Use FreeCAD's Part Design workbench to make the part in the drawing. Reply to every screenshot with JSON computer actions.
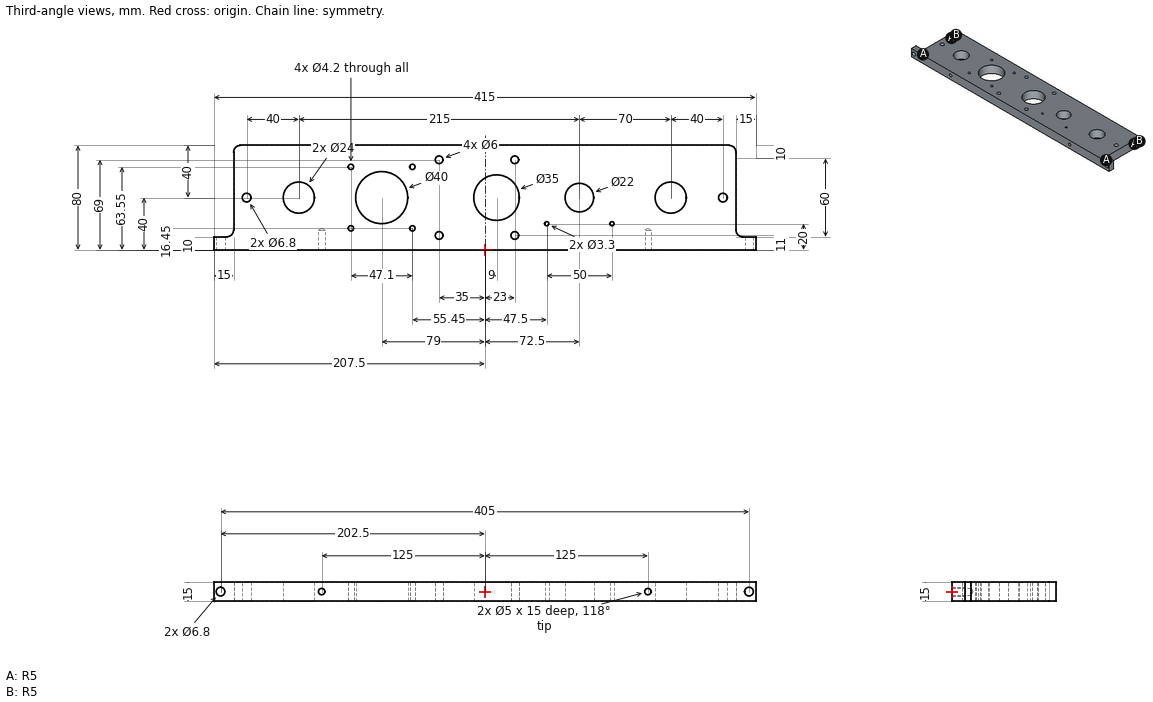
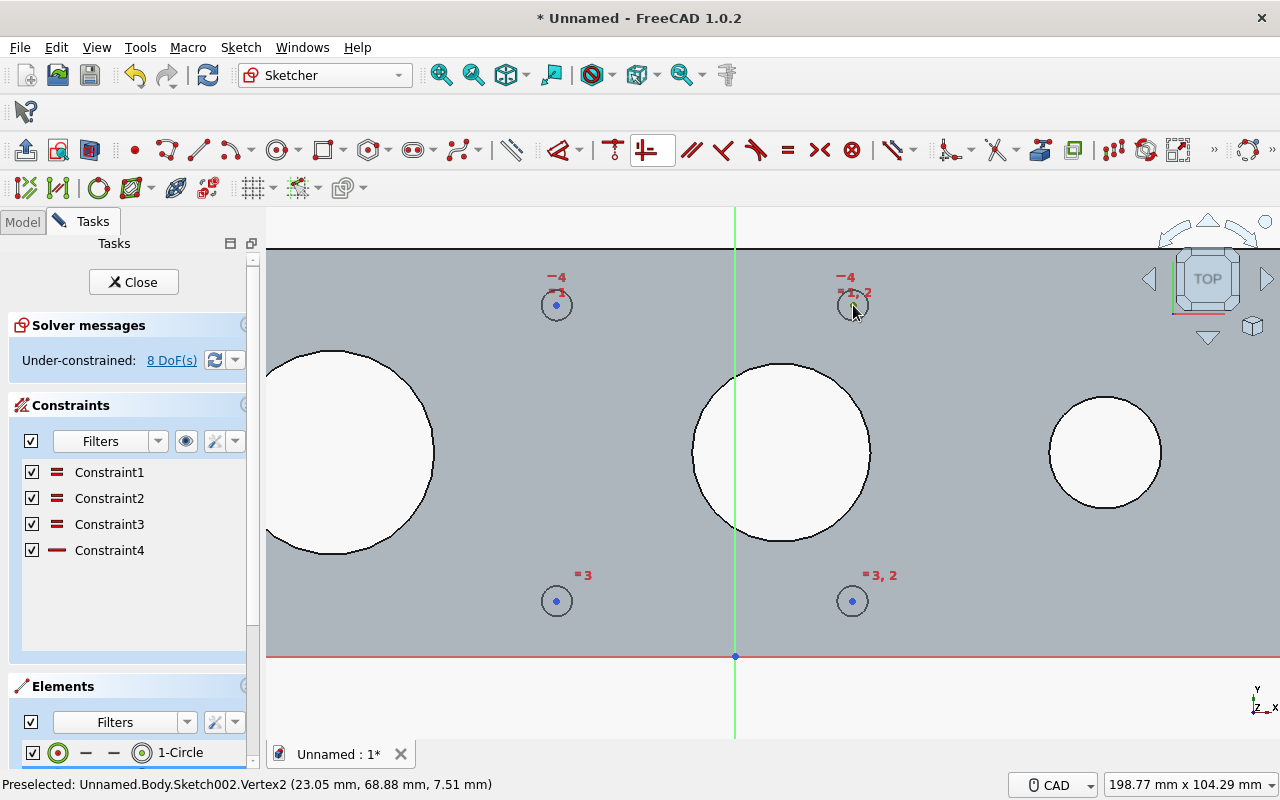
{"action": "left_click", "coordinate": [853, 601]}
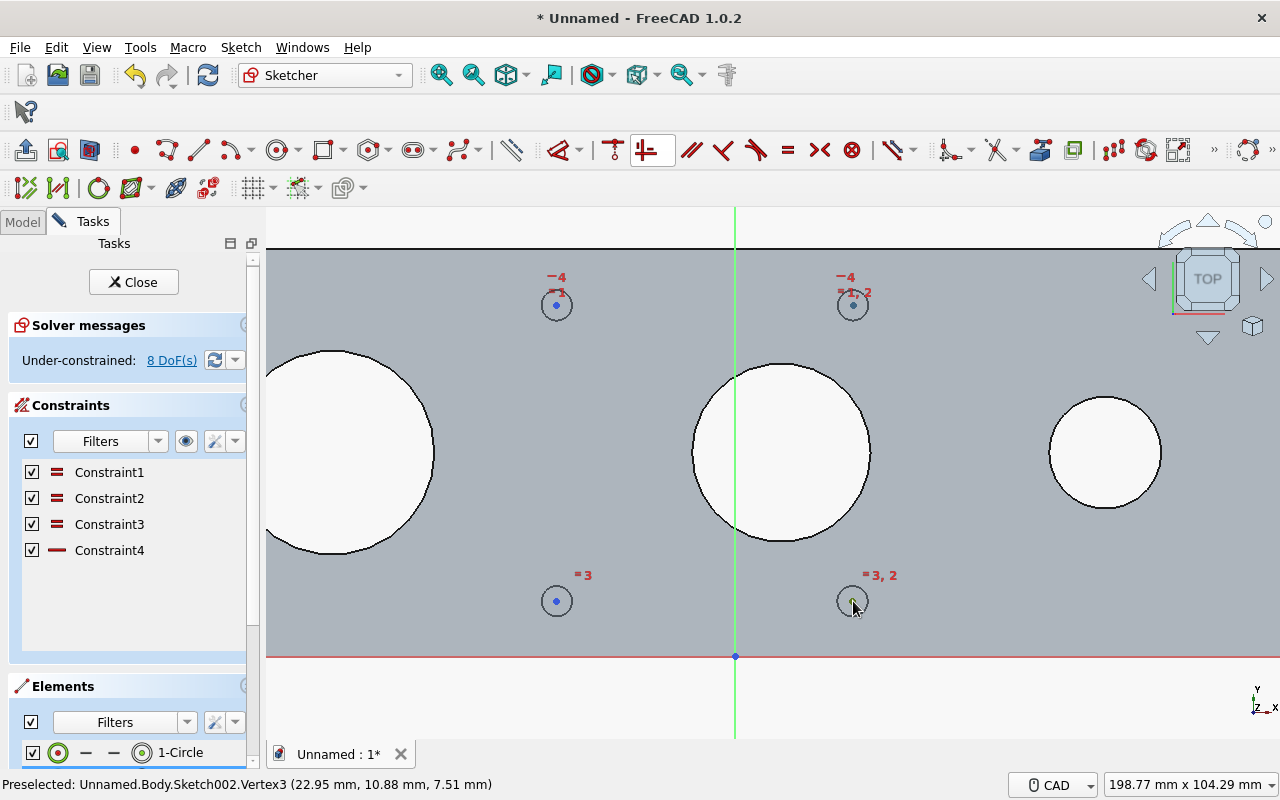
{"action": "left_click", "coordinate": [670, 150]}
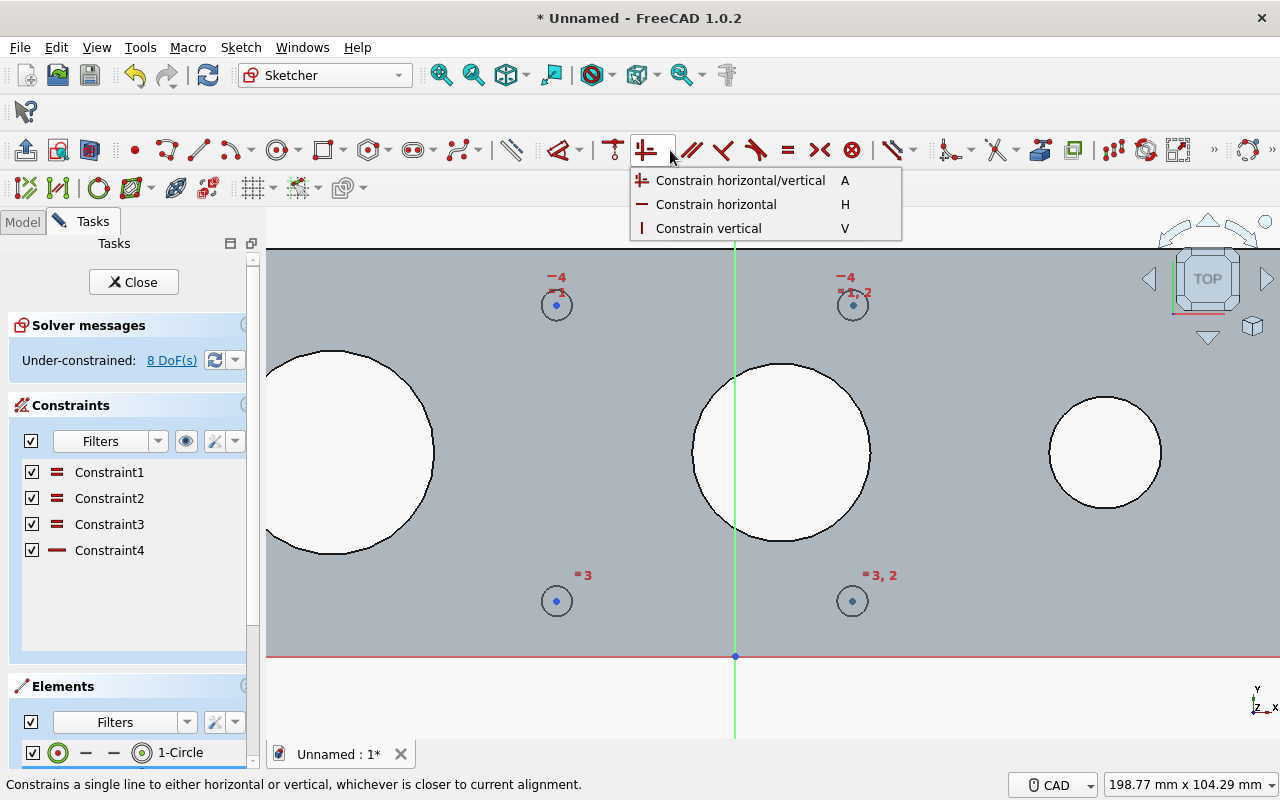
{"action": "left_click", "coordinate": [766, 228]}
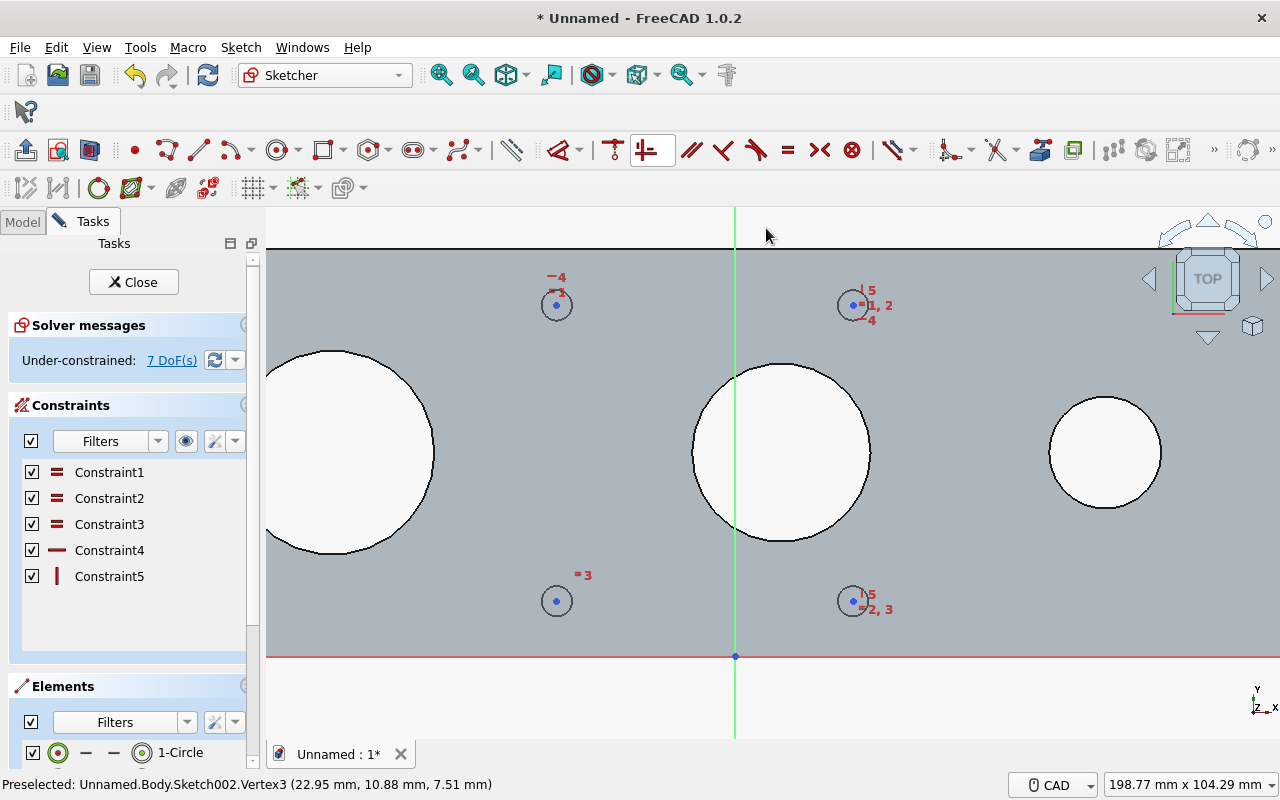
{"action": "left_click", "coordinate": [557, 305]}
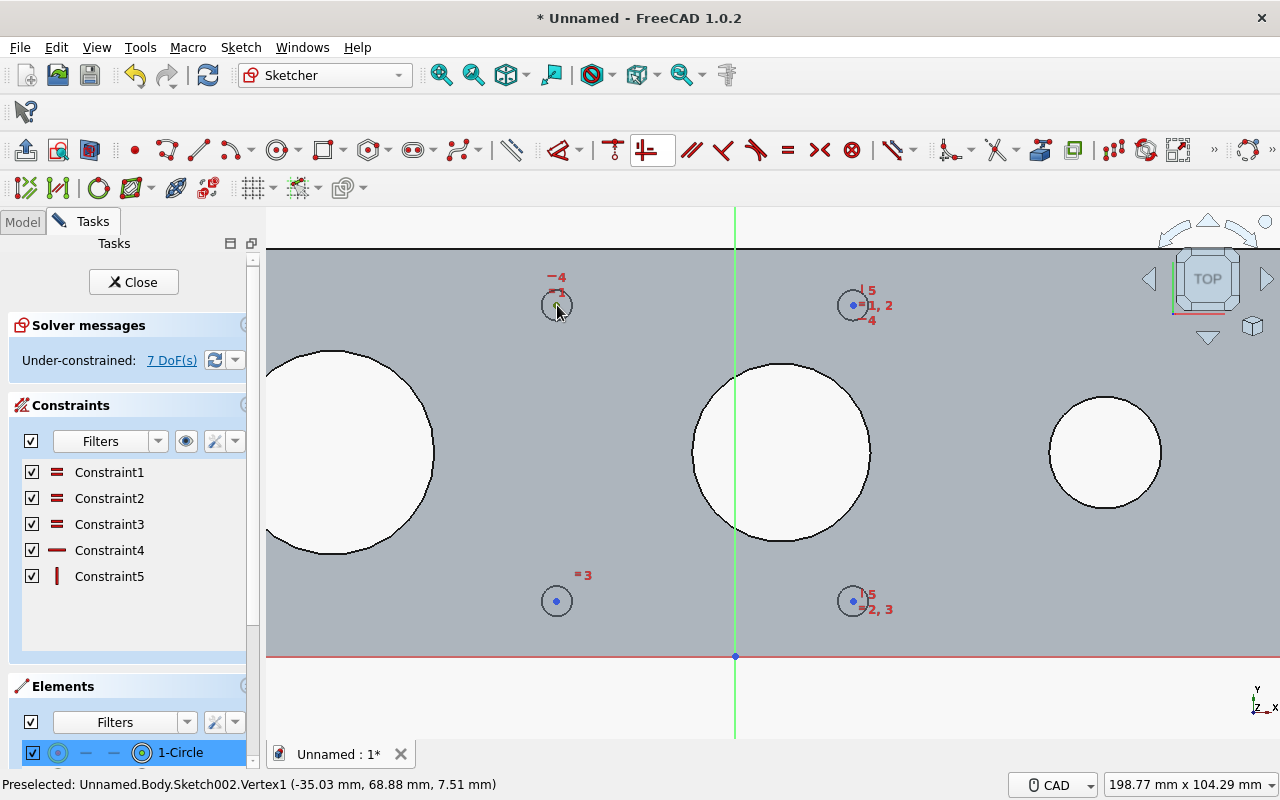
{"action": "left_click", "coordinate": [557, 601]}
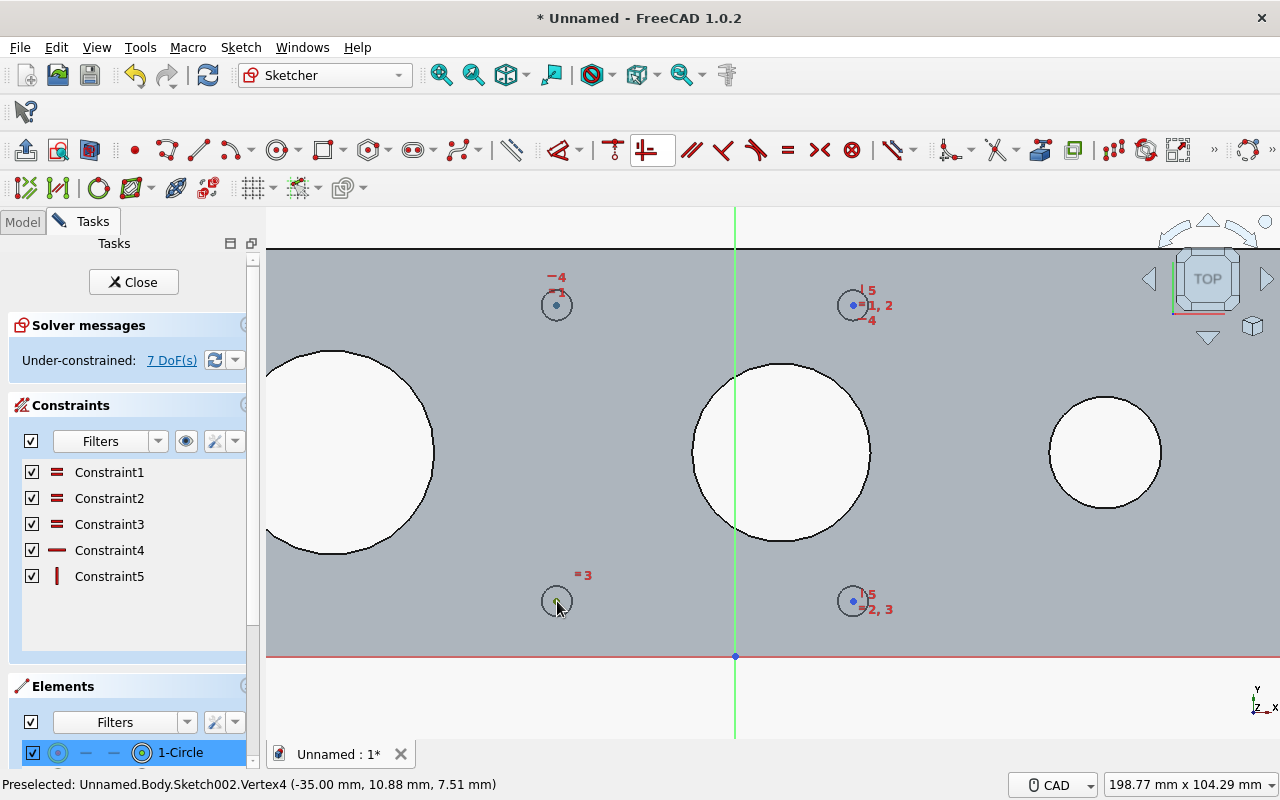
{"action": "key", "text": "v"}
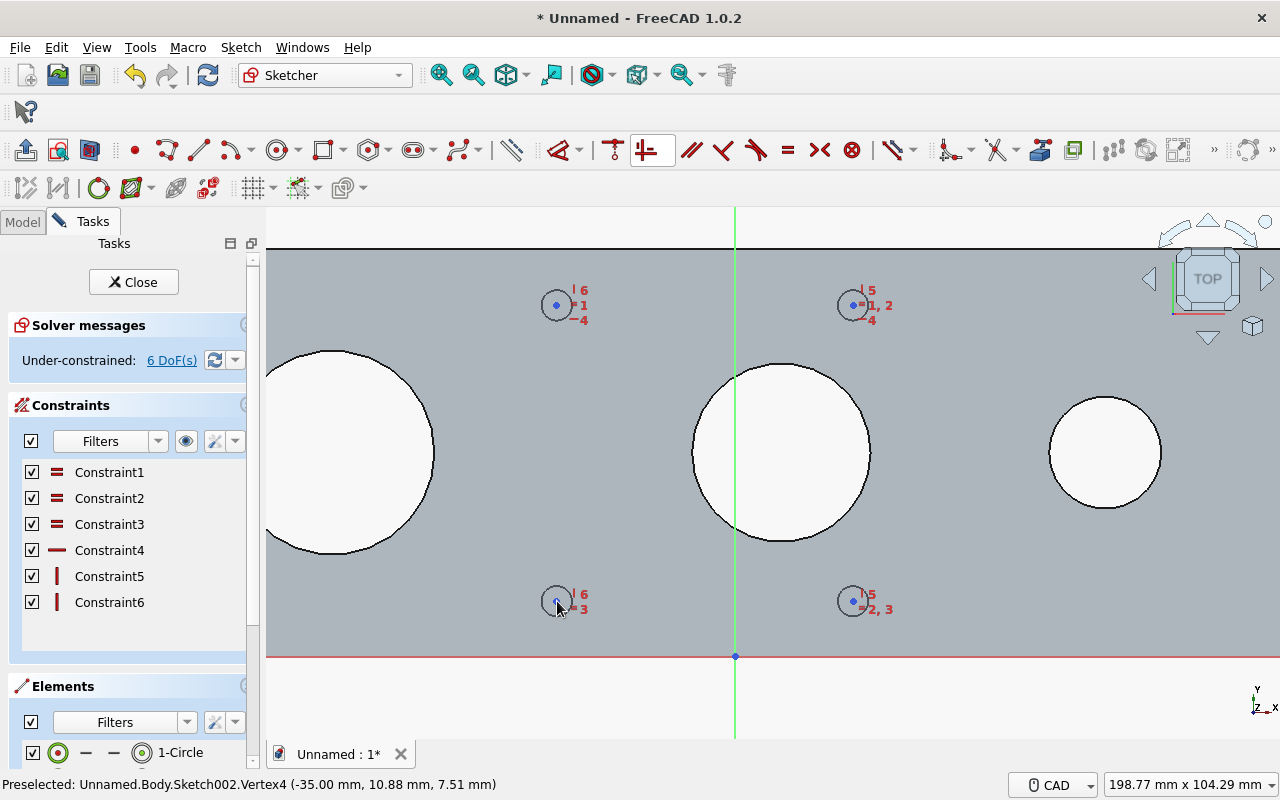
{"action": "left_click", "coordinate": [853, 601]}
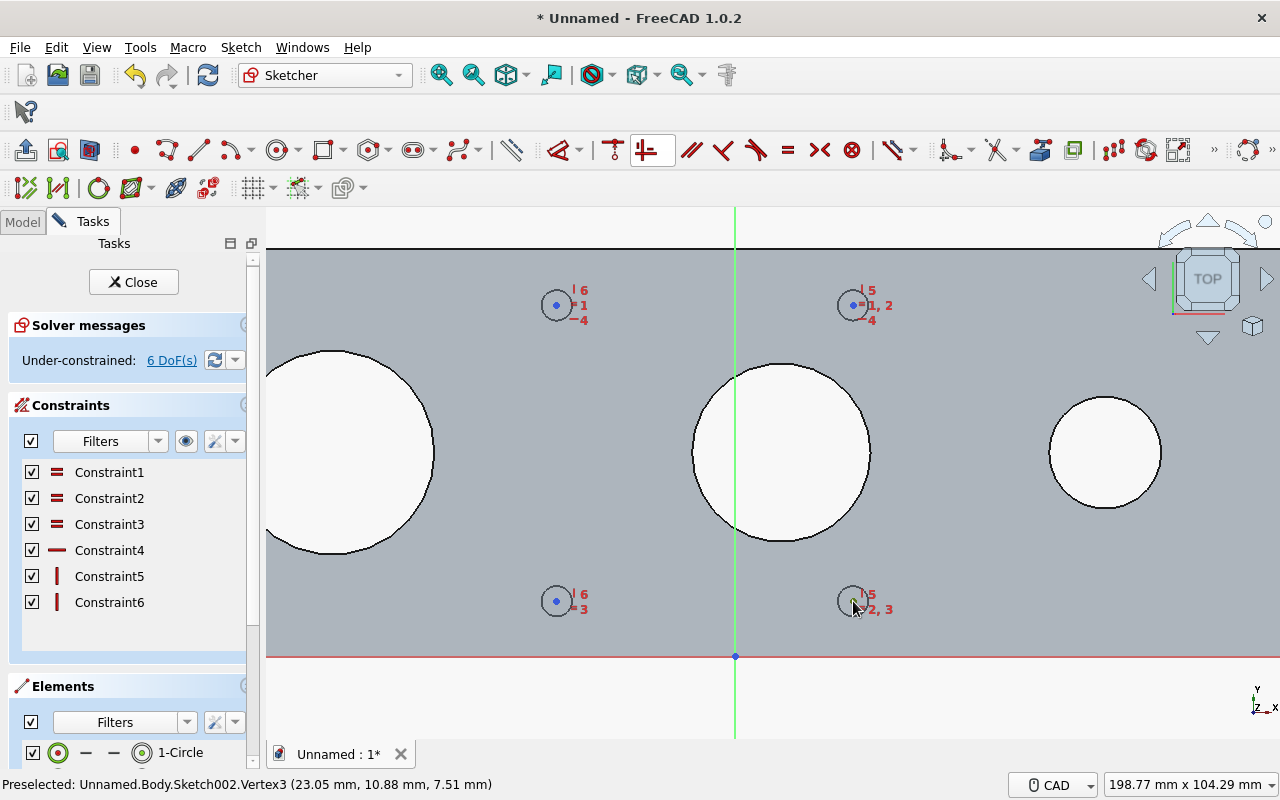
{"action": "left_click", "coordinate": [557, 601]}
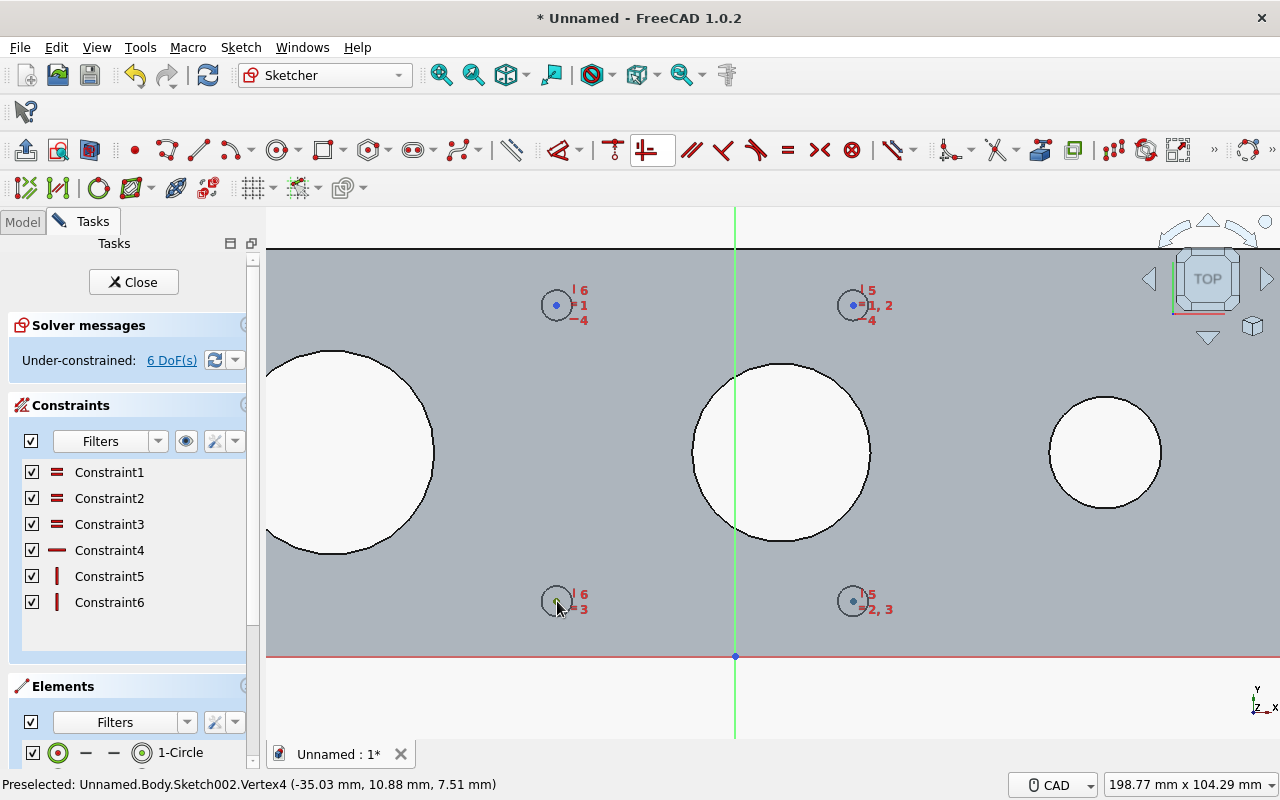
{"action": "left_click", "coordinate": [670, 150]}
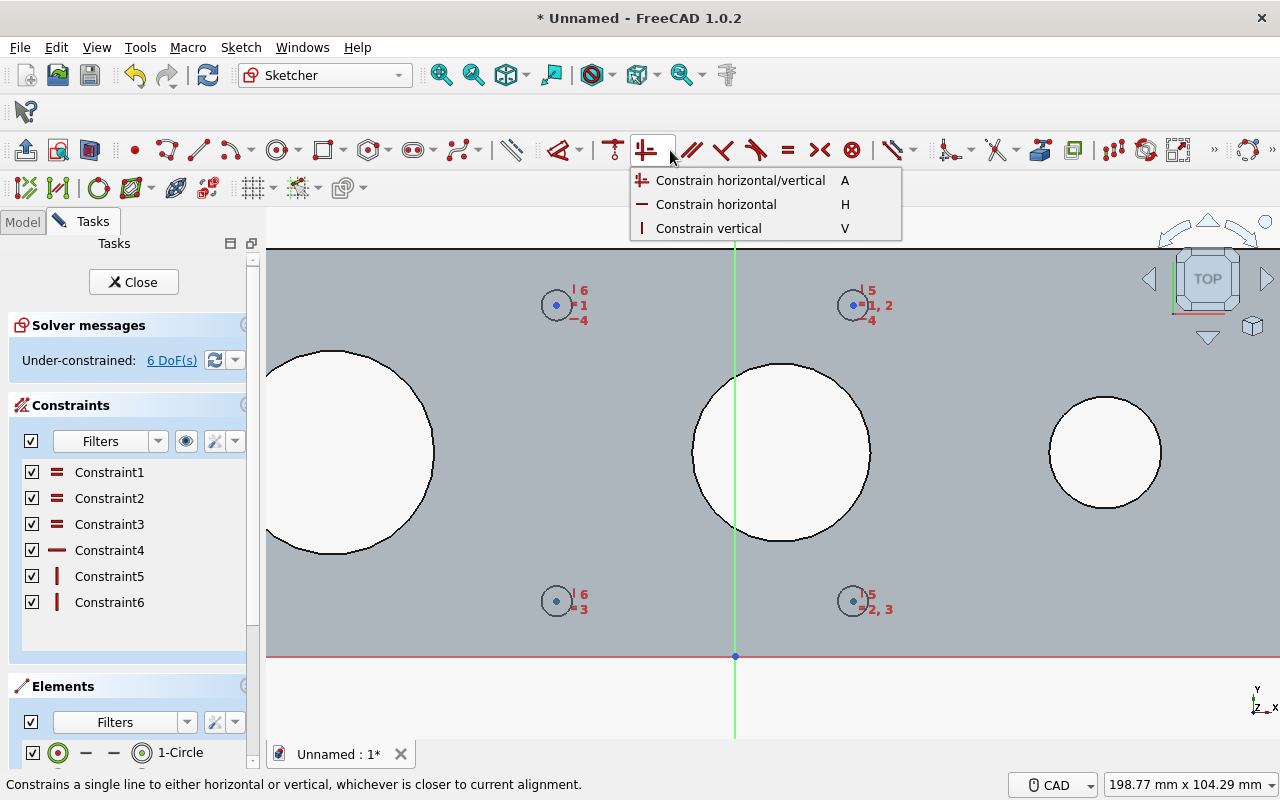
{"action": "left_click", "coordinate": [766, 204]}